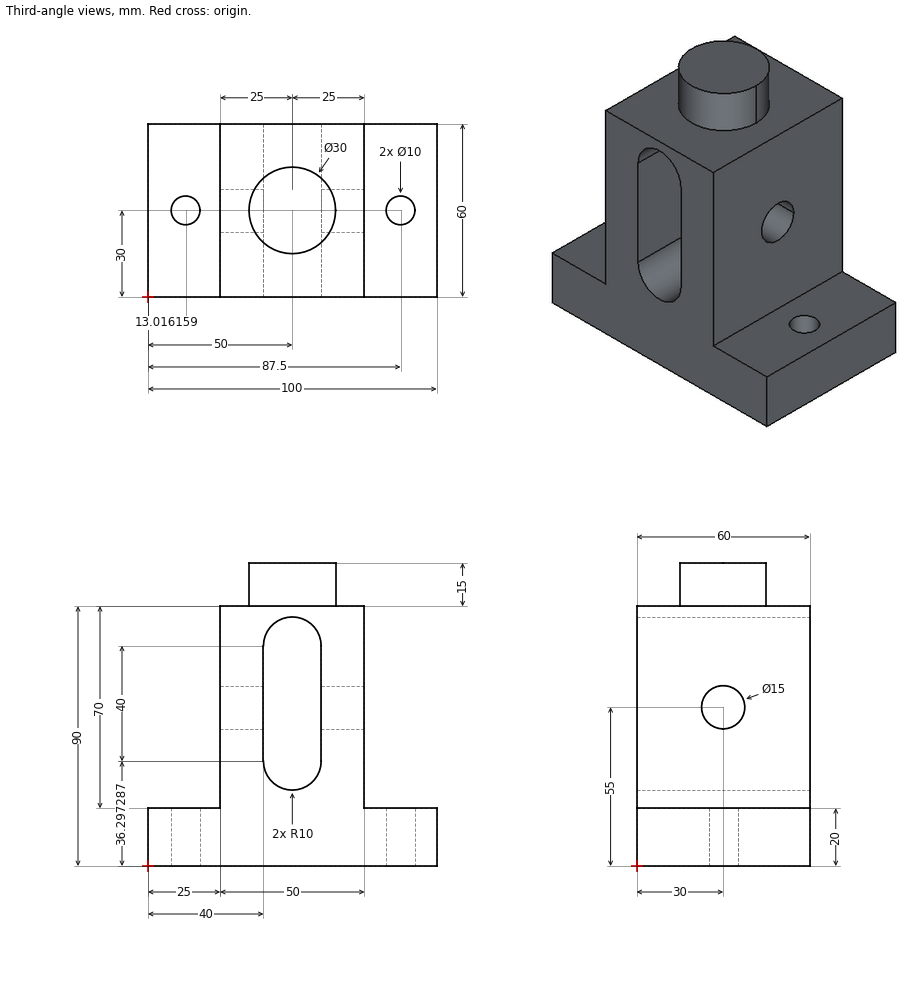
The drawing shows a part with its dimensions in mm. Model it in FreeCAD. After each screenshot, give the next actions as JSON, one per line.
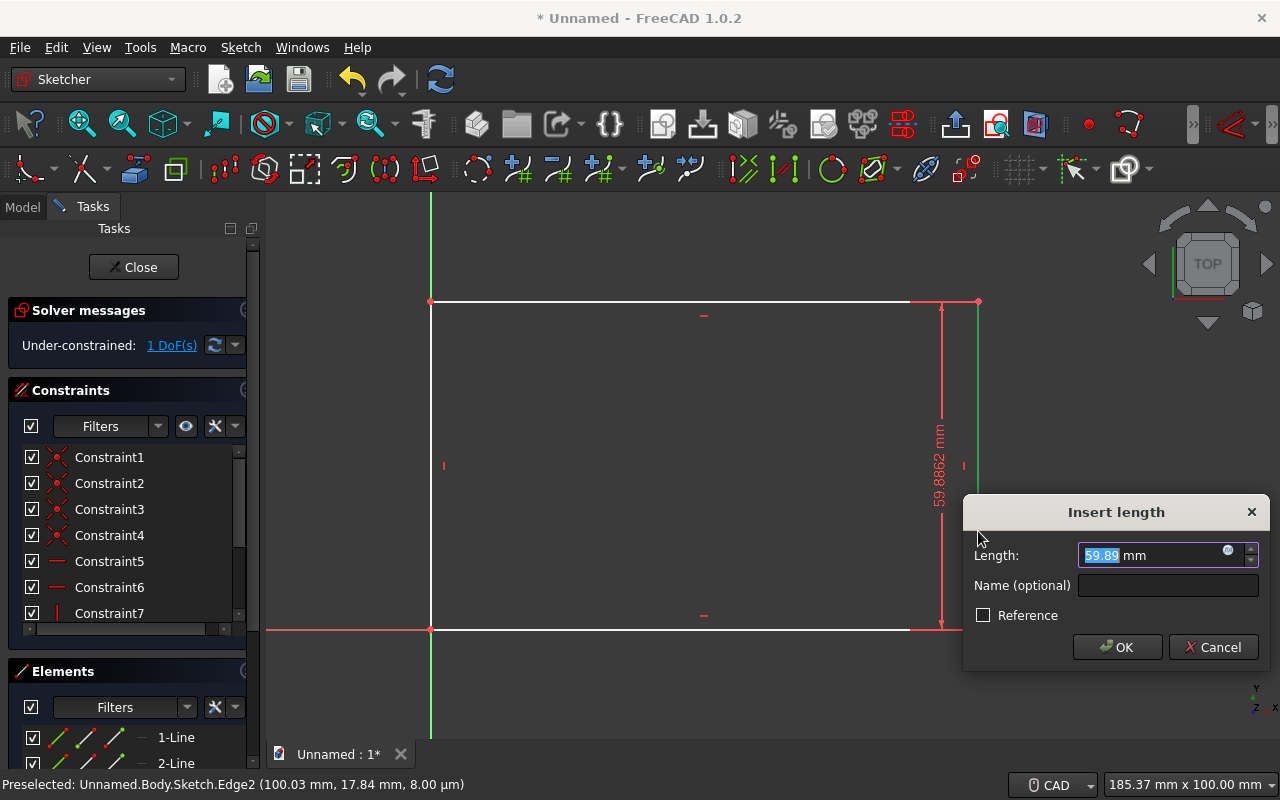
{"action": "type", "text": "60"}
{"action": "key", "text": "Return"}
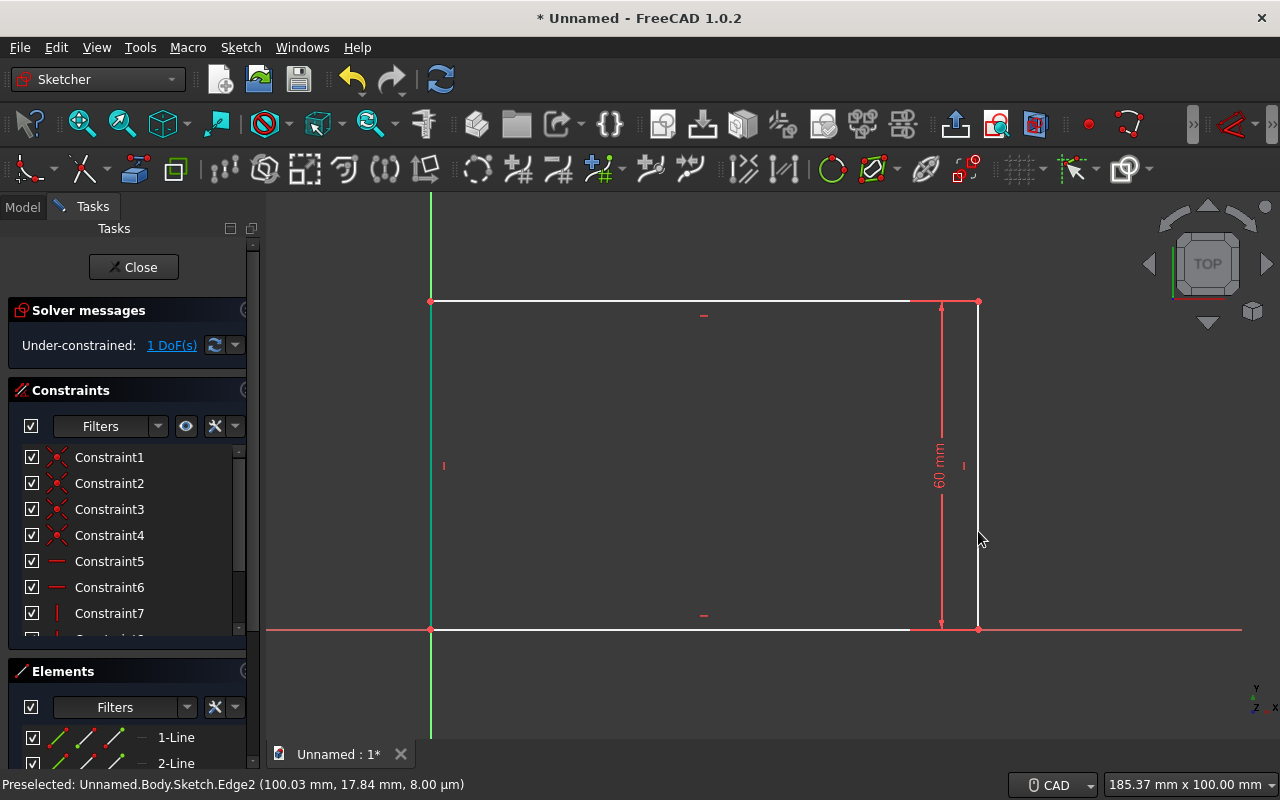
{"action": "left_click", "coordinate": [595, 630]}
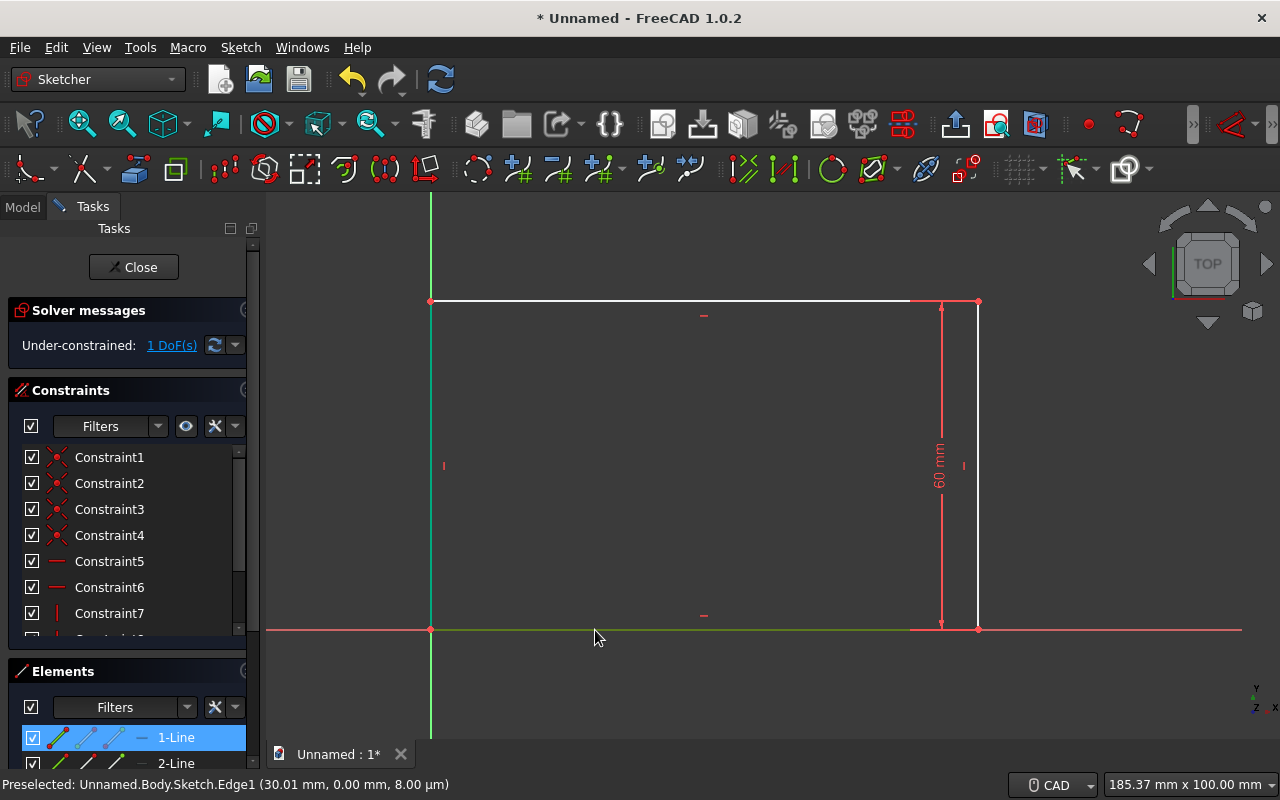
{"action": "key", "text": "l"}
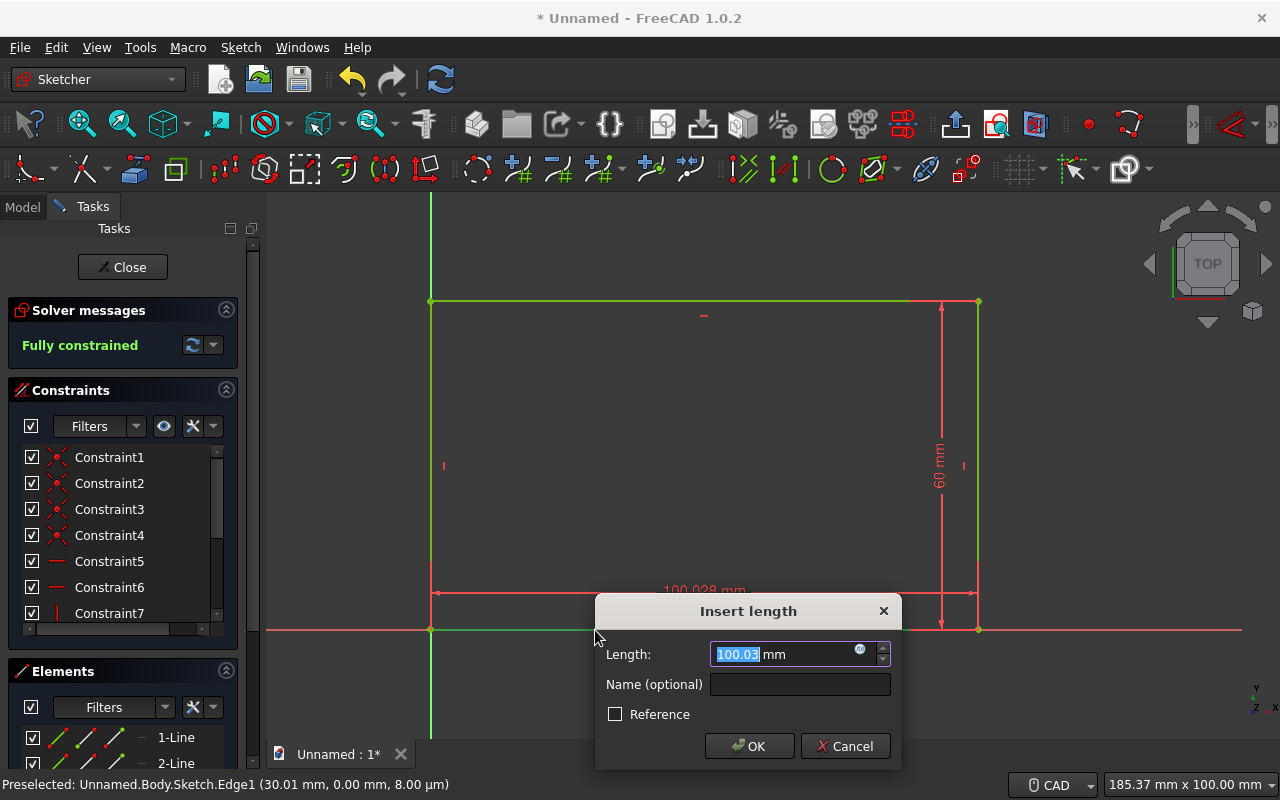
{"action": "type", "text": "100"}
{"action": "key", "text": "Return"}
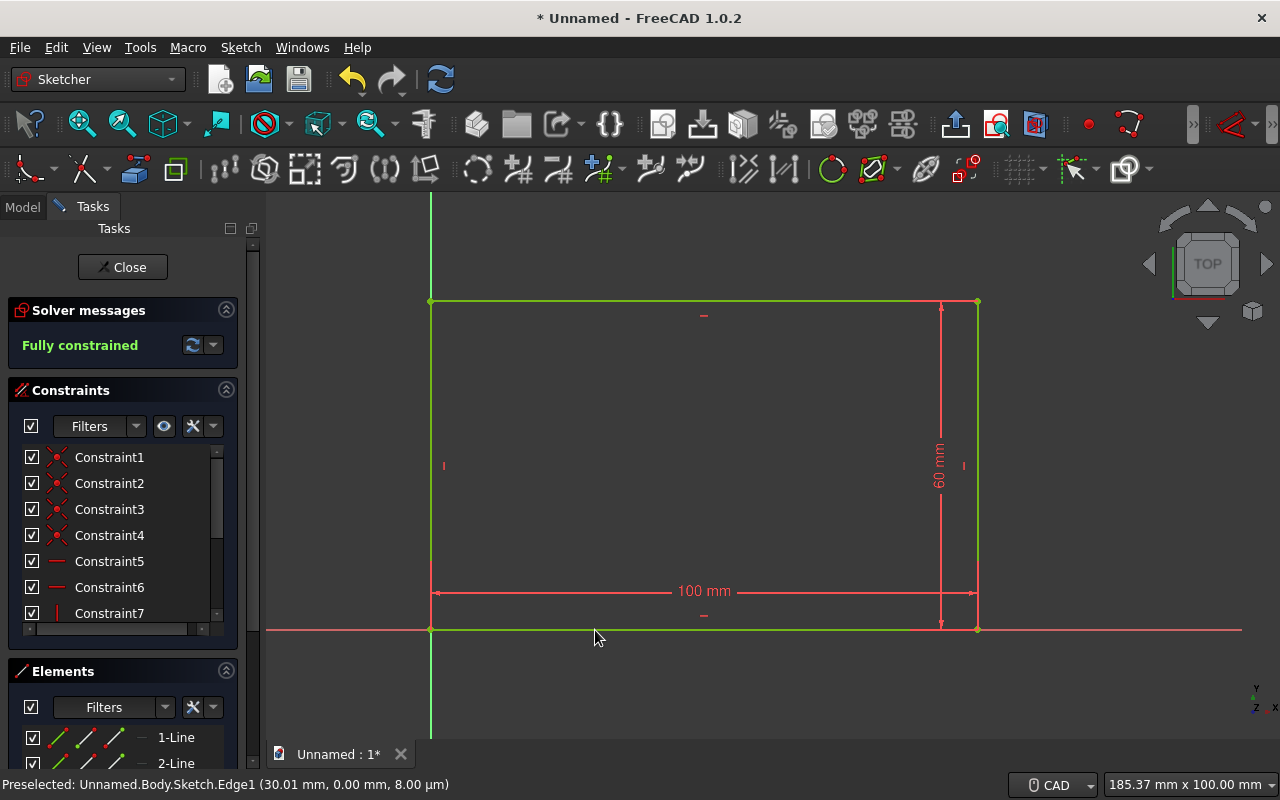
{"action": "left_click", "coordinate": [123, 267]}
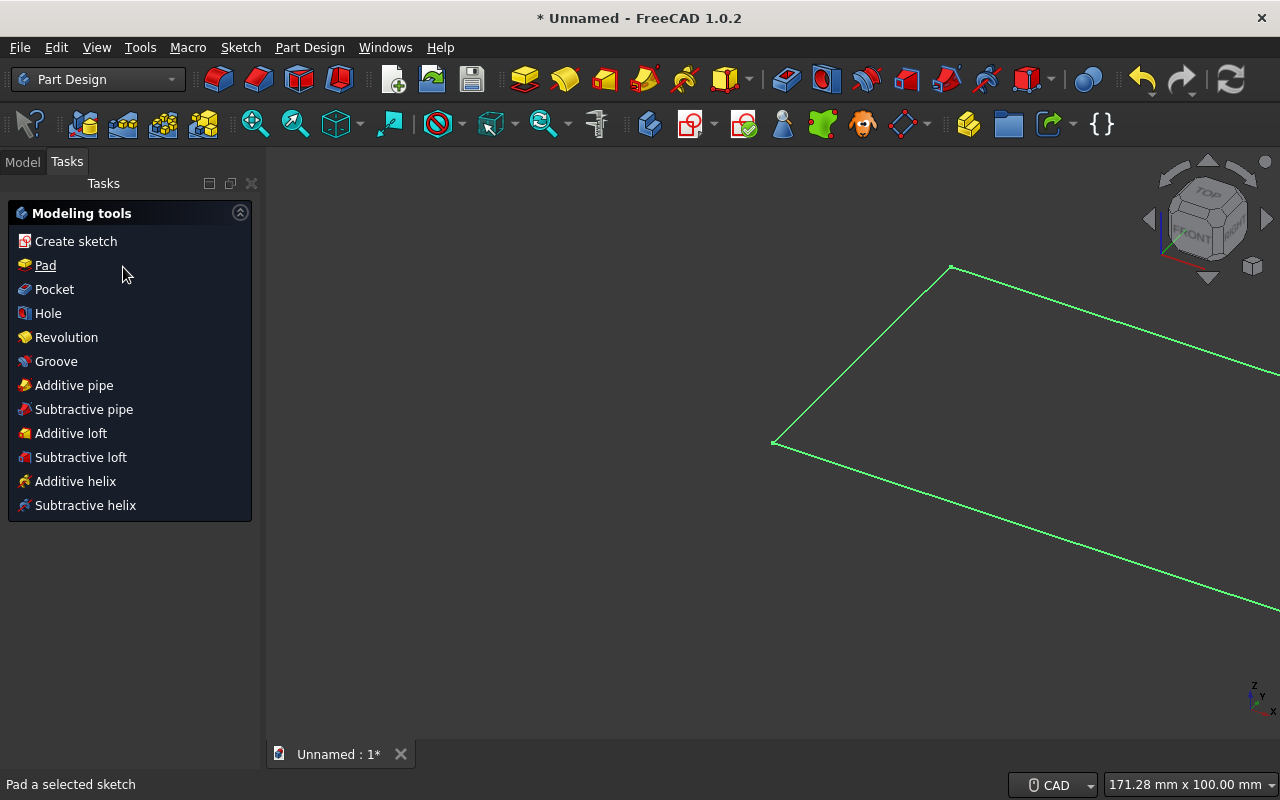
{"action": "left_click", "coordinate": [526, 80]}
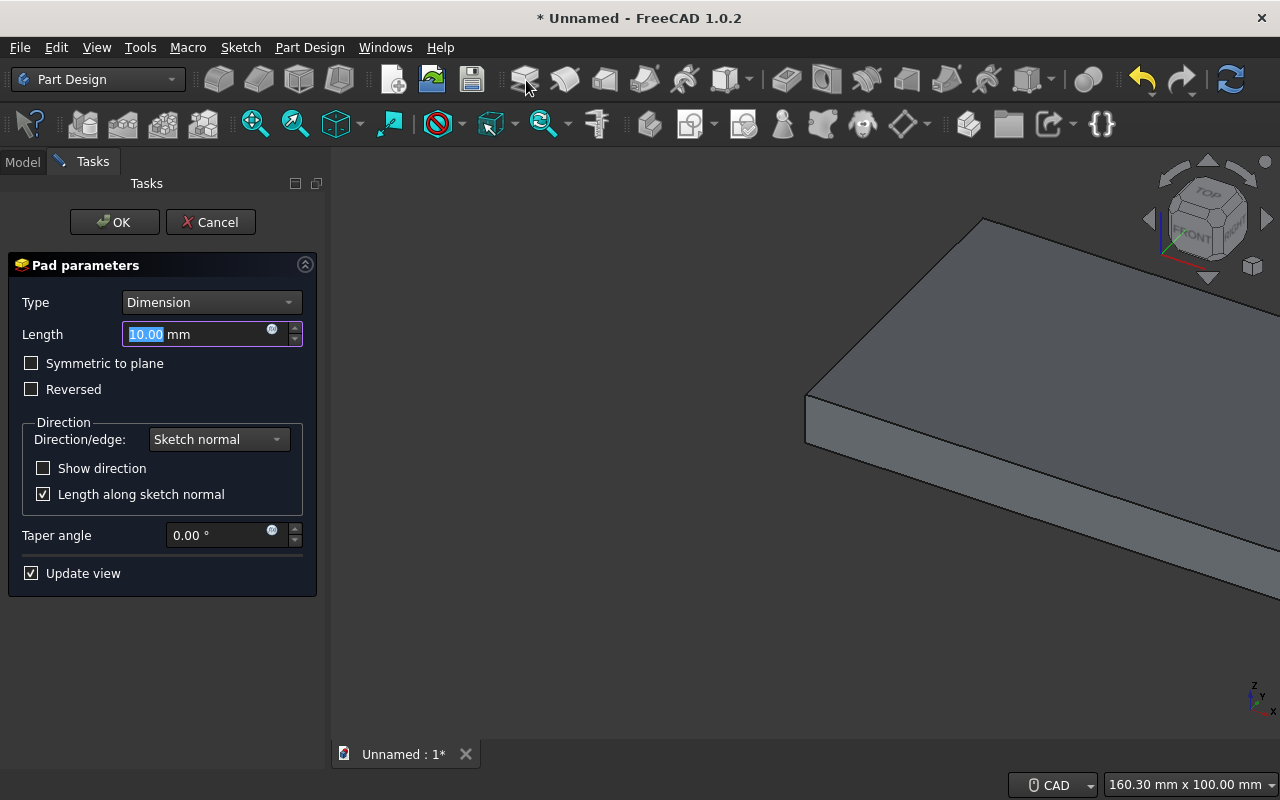
{"action": "type", "text": "20"}
{"action": "key", "text": "Tab"}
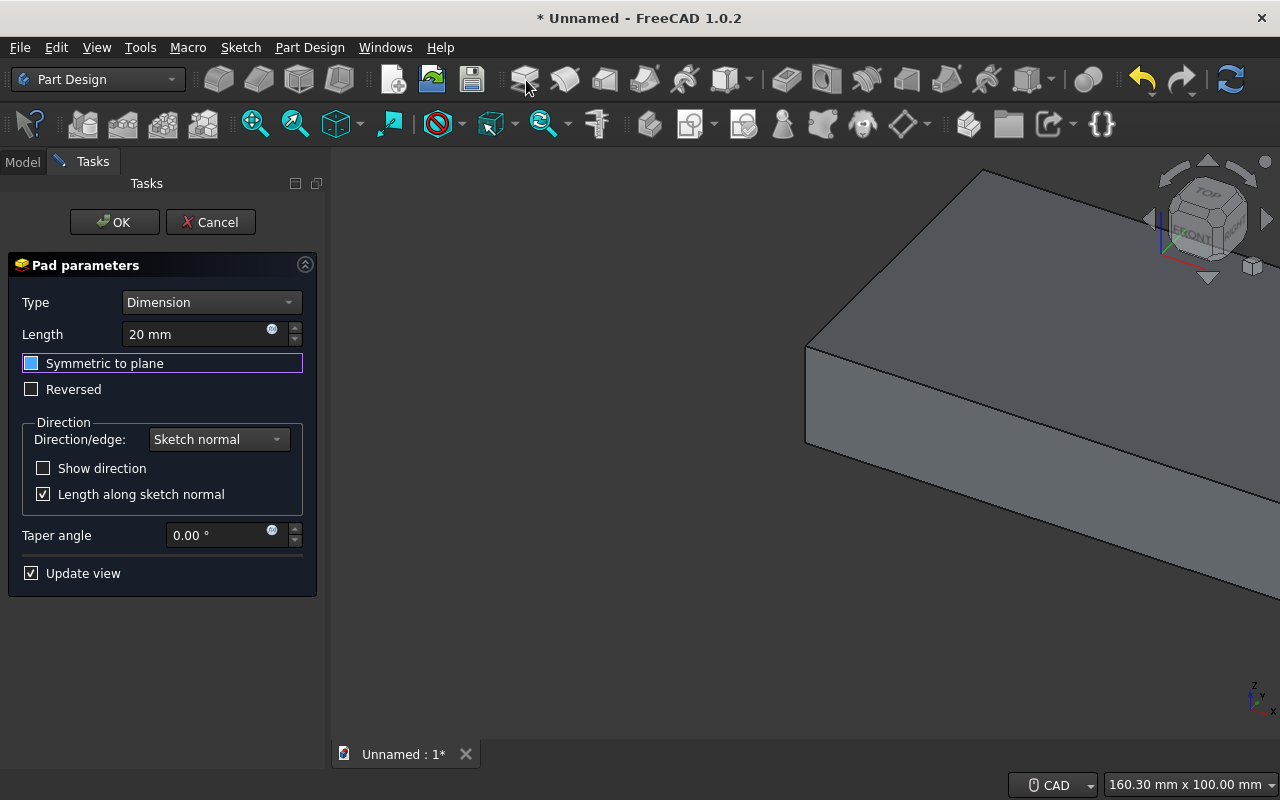
{"action": "left_click", "coordinate": [115, 222]}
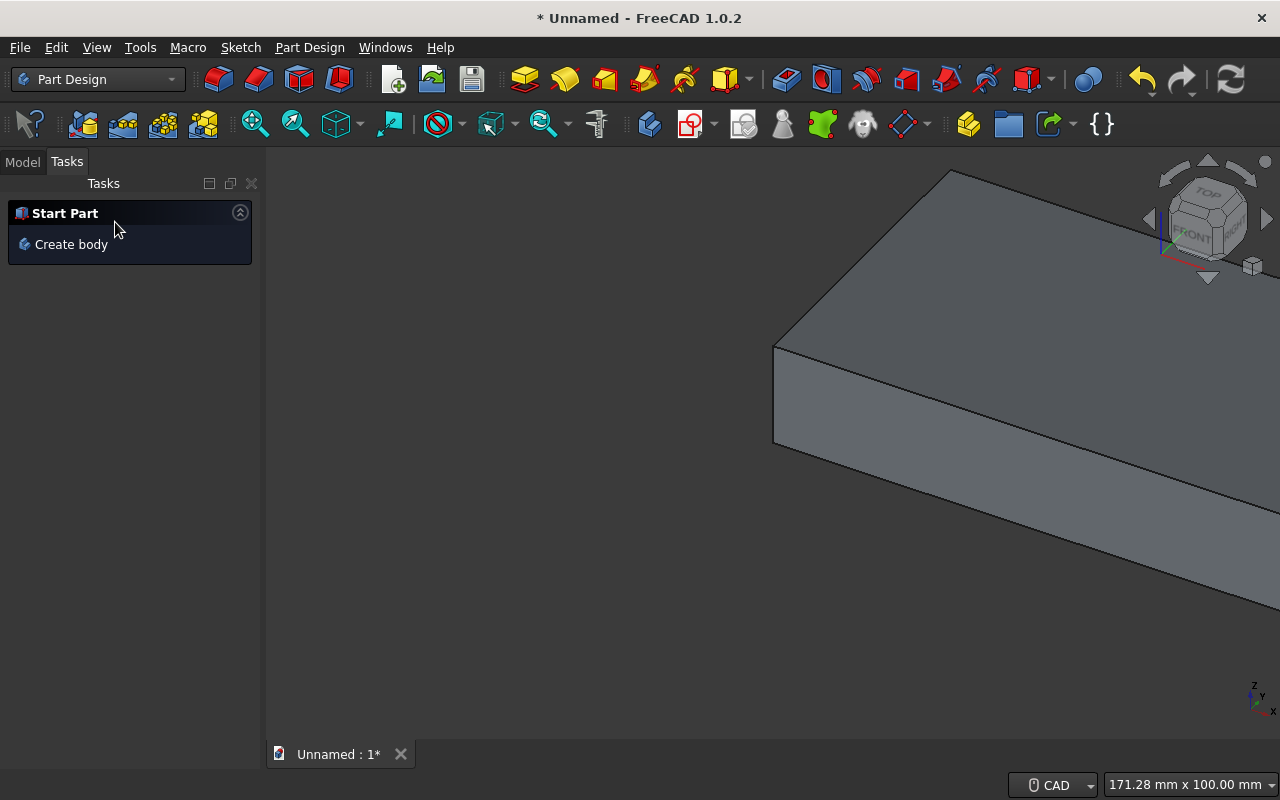
{"action": "key", "text": "v f"}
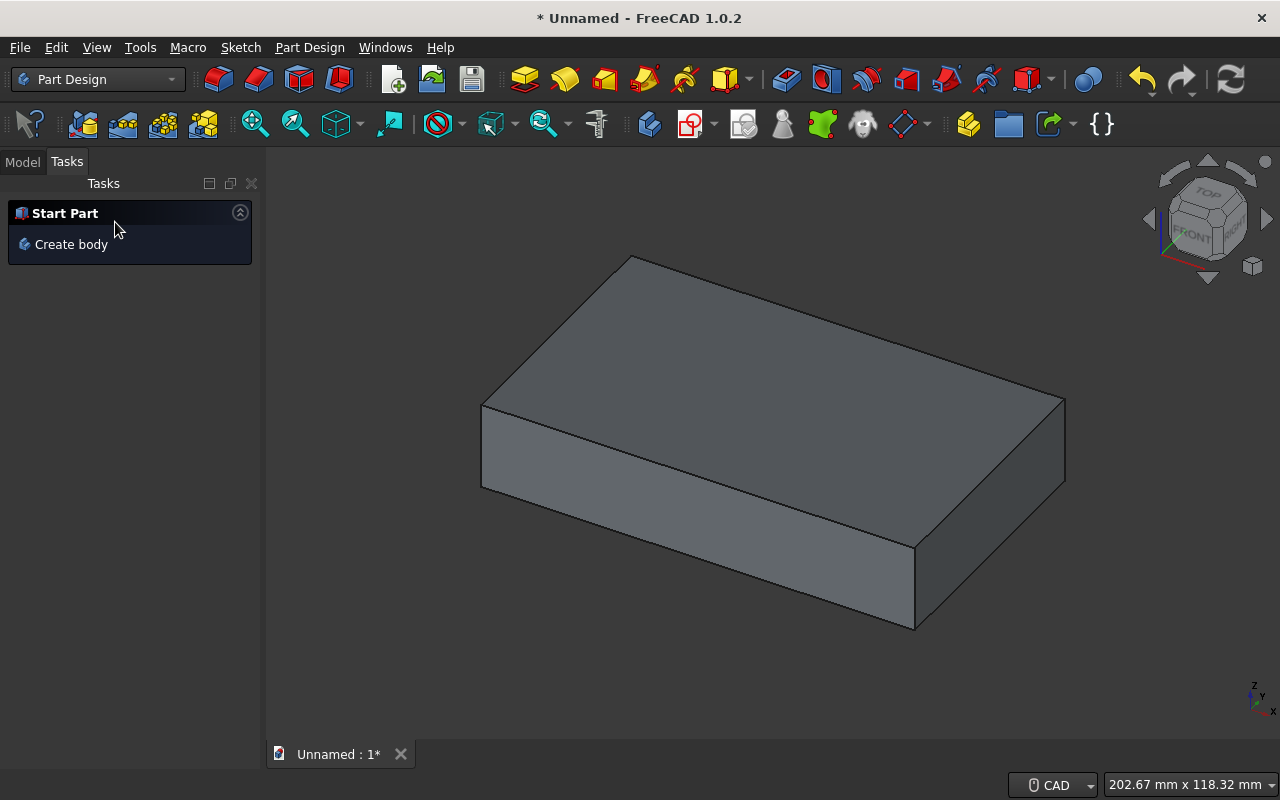
{"action": "left_click", "coordinate": [690, 124]}